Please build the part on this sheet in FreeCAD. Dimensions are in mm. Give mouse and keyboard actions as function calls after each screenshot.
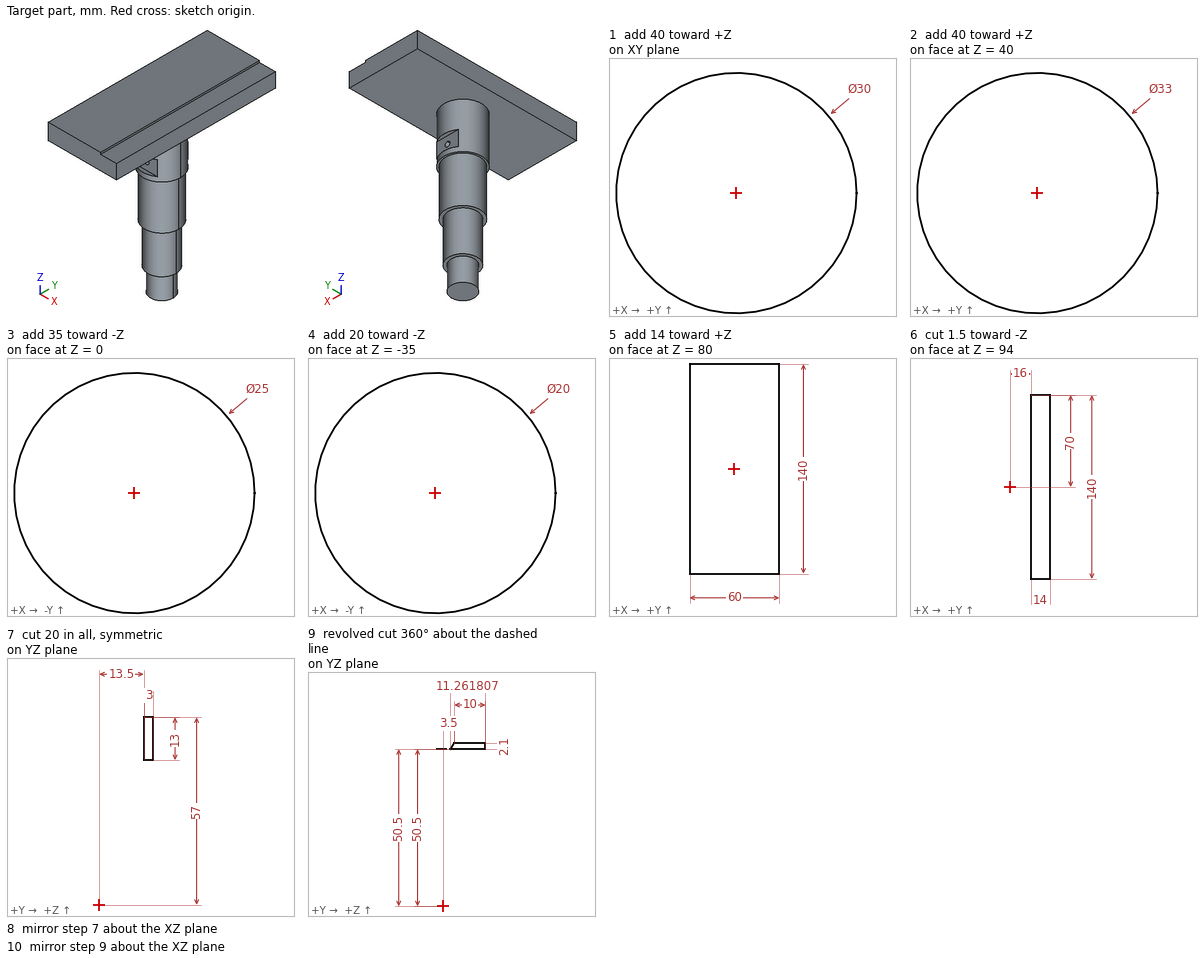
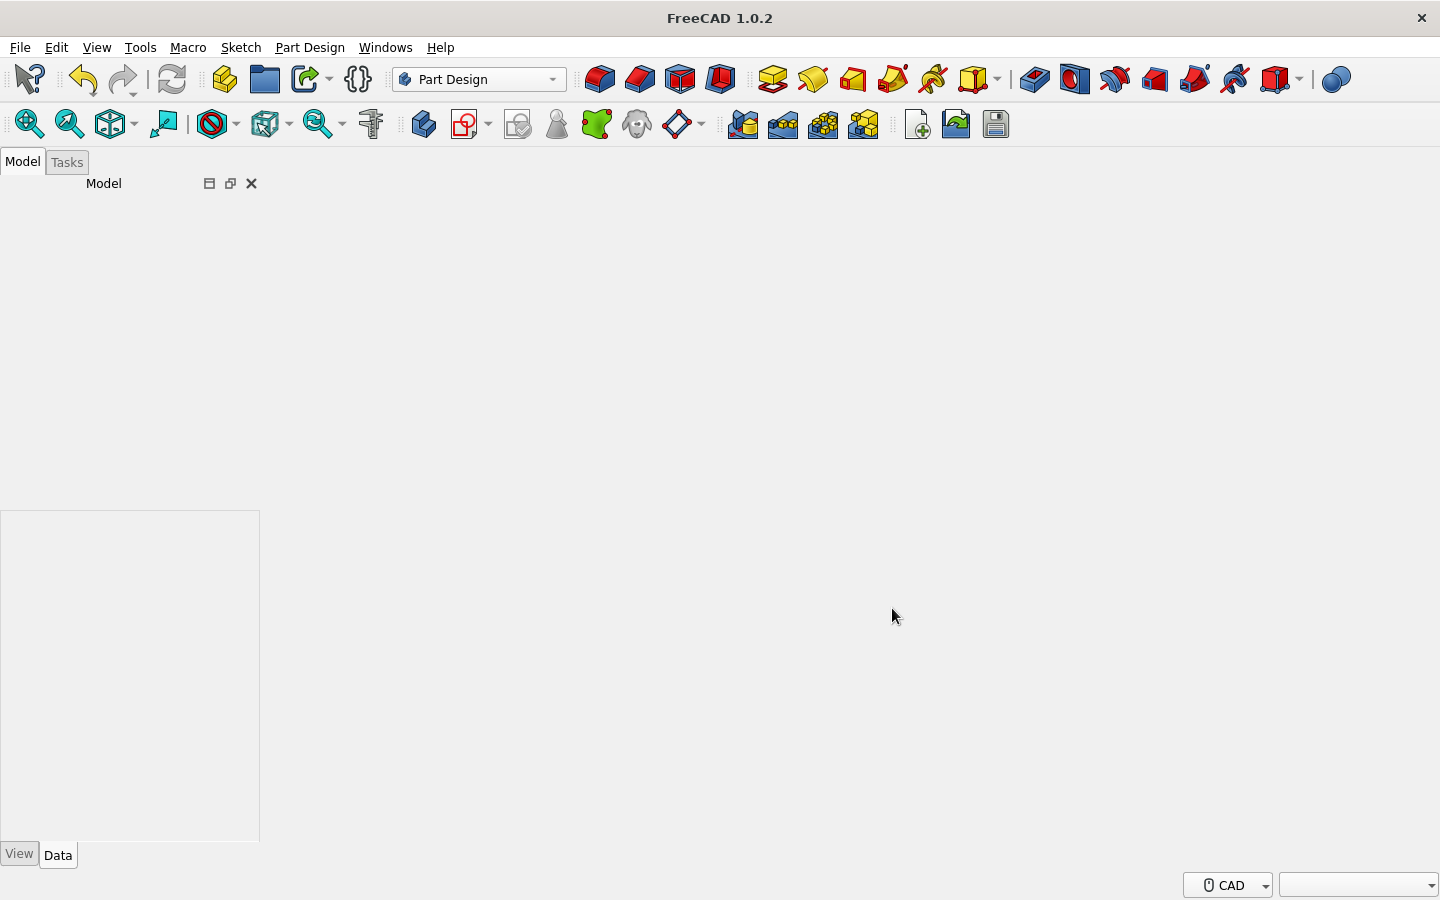
click(916, 124)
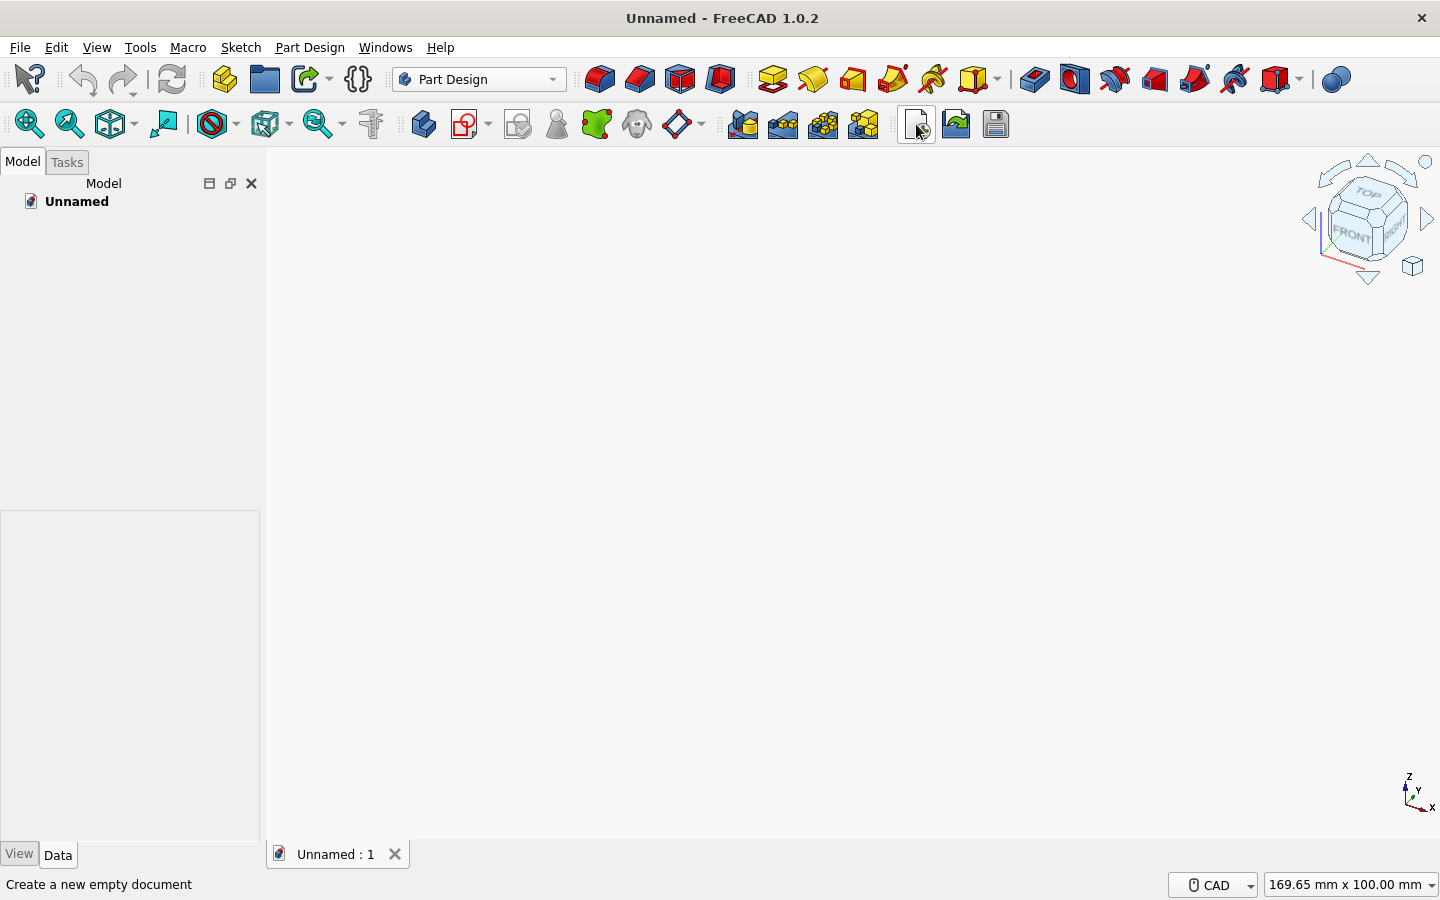
click(464, 124)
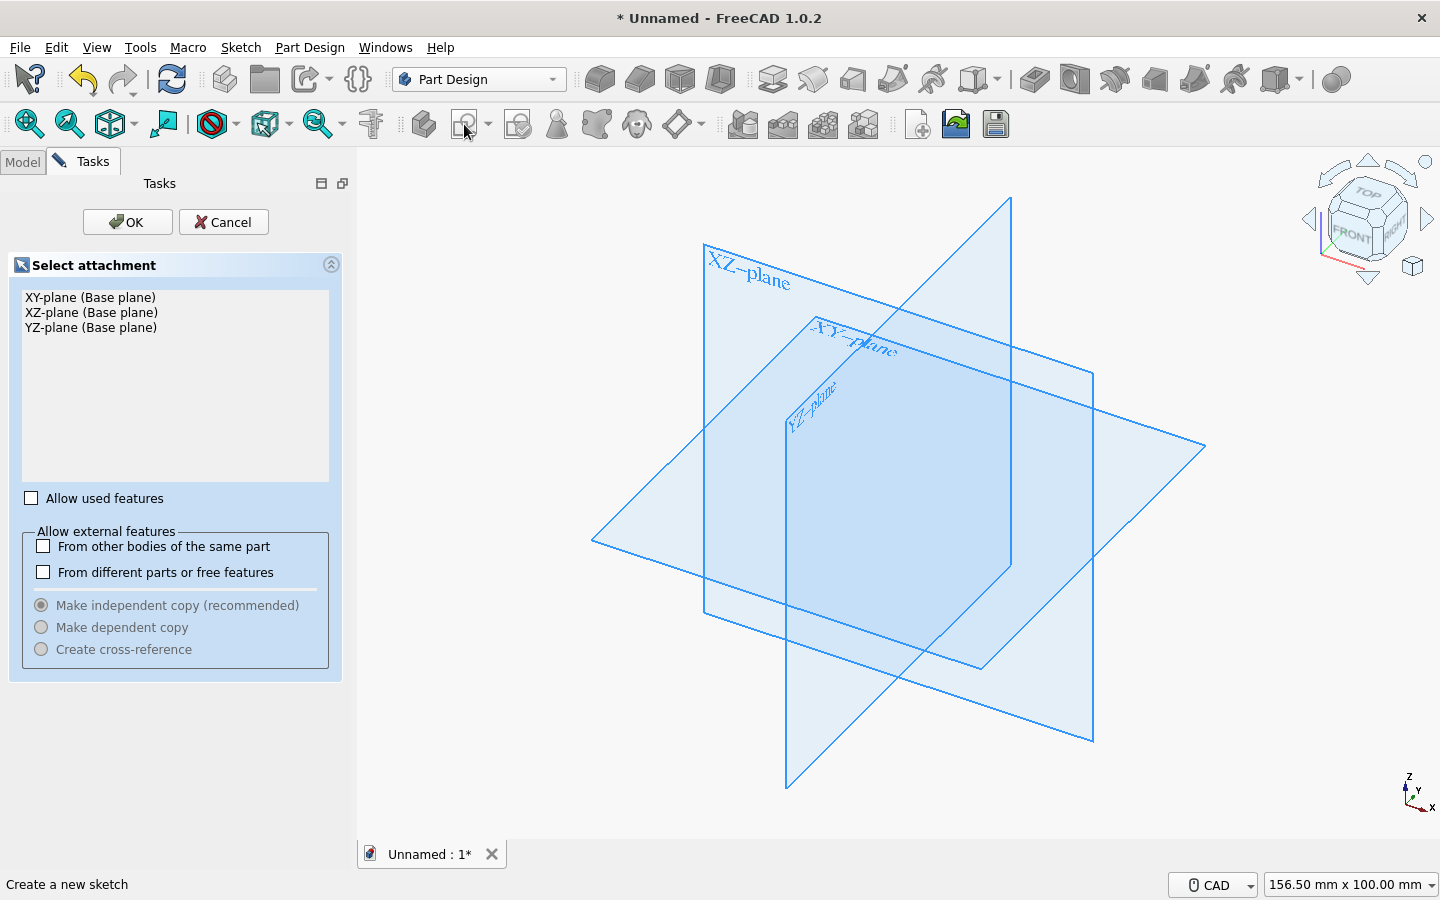
click(82, 298)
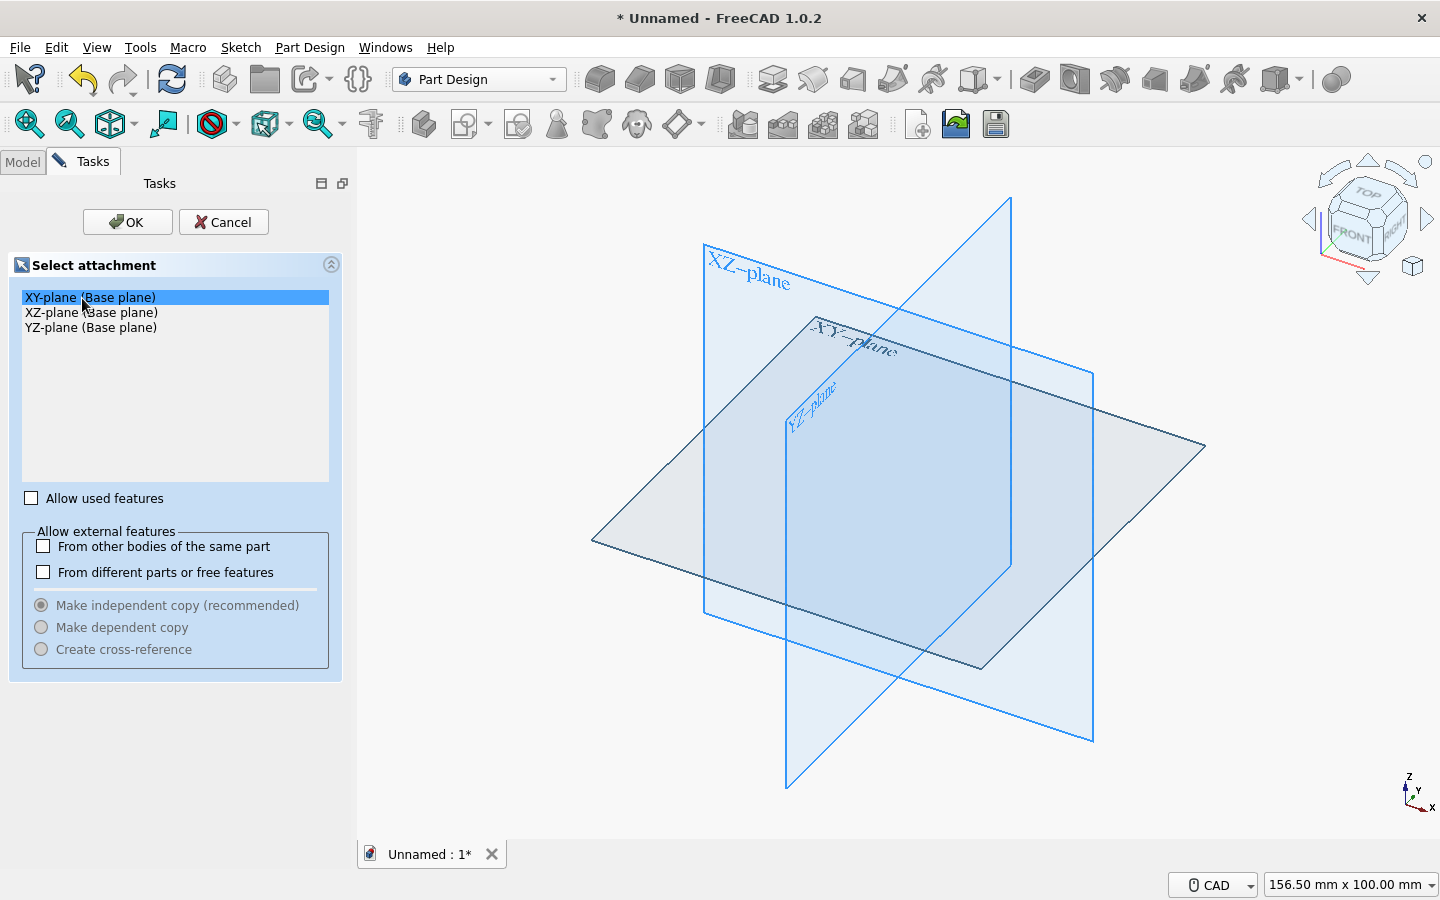
click(128, 222)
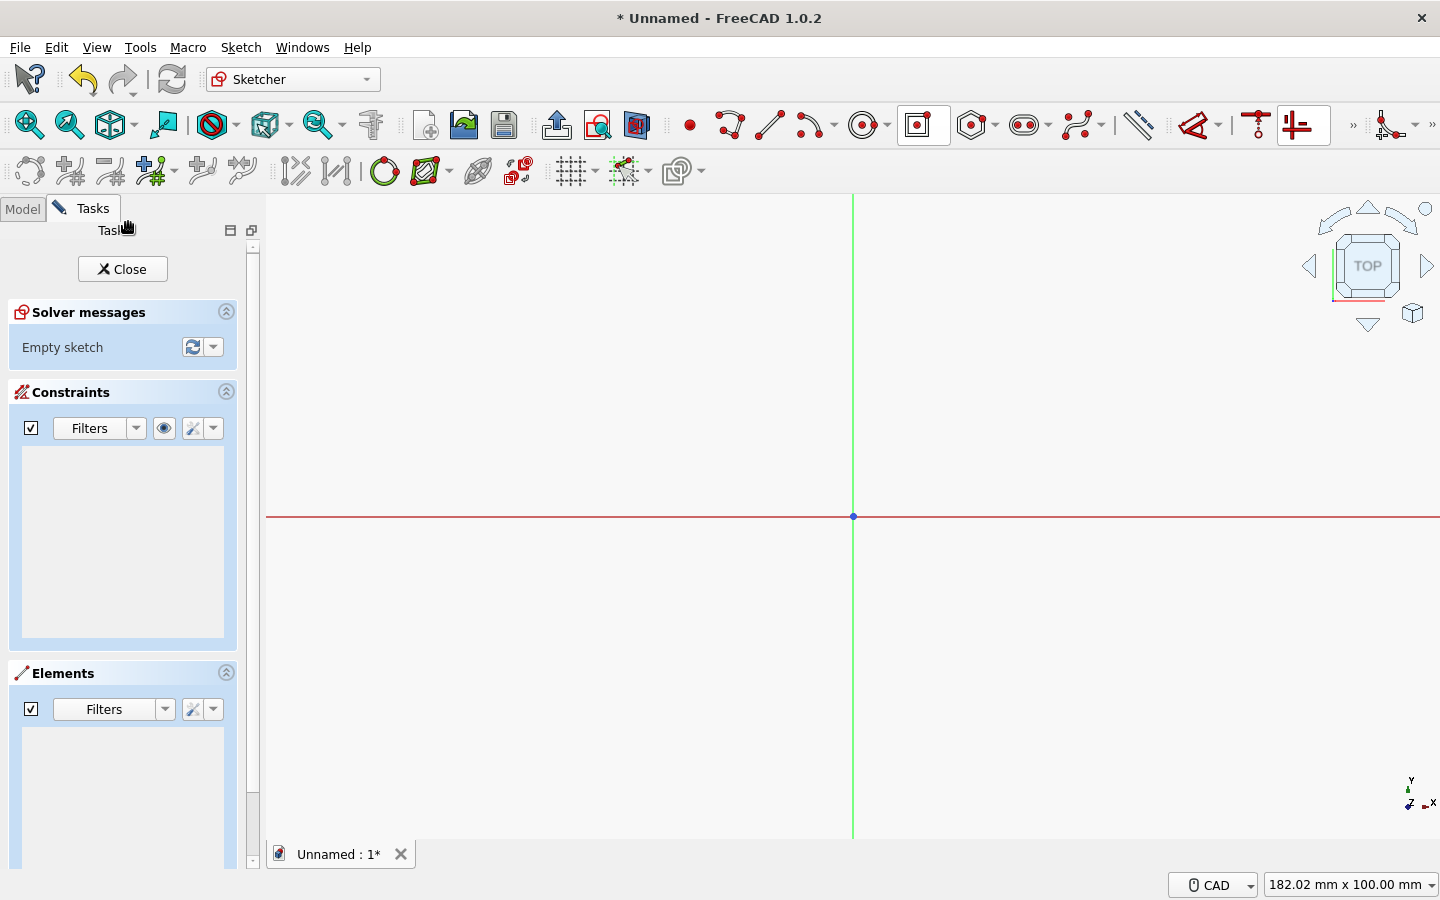
scroll(909, 517, up, 4)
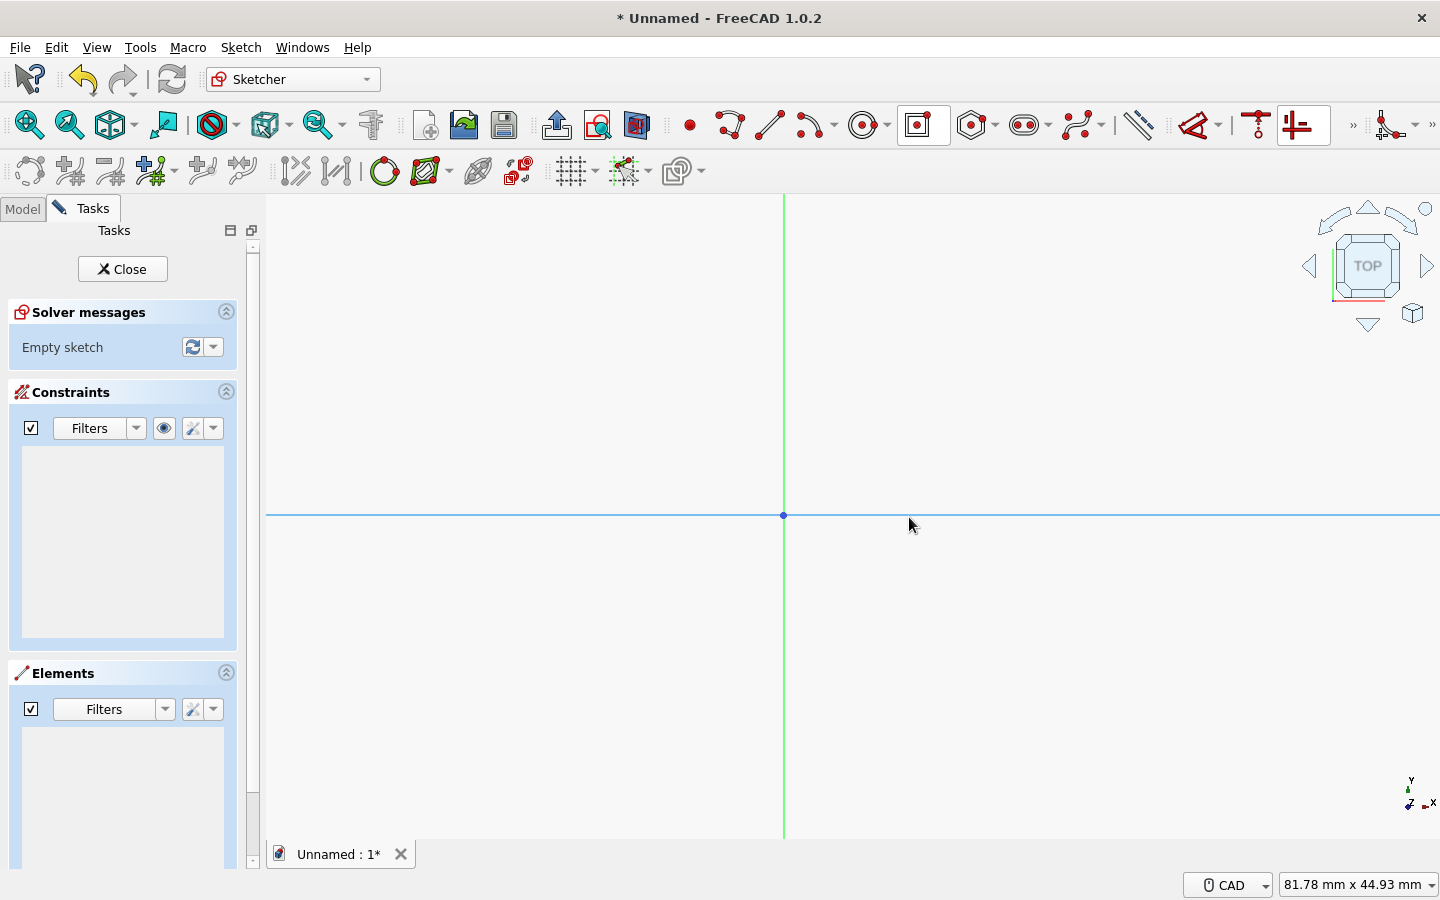
click(864, 126)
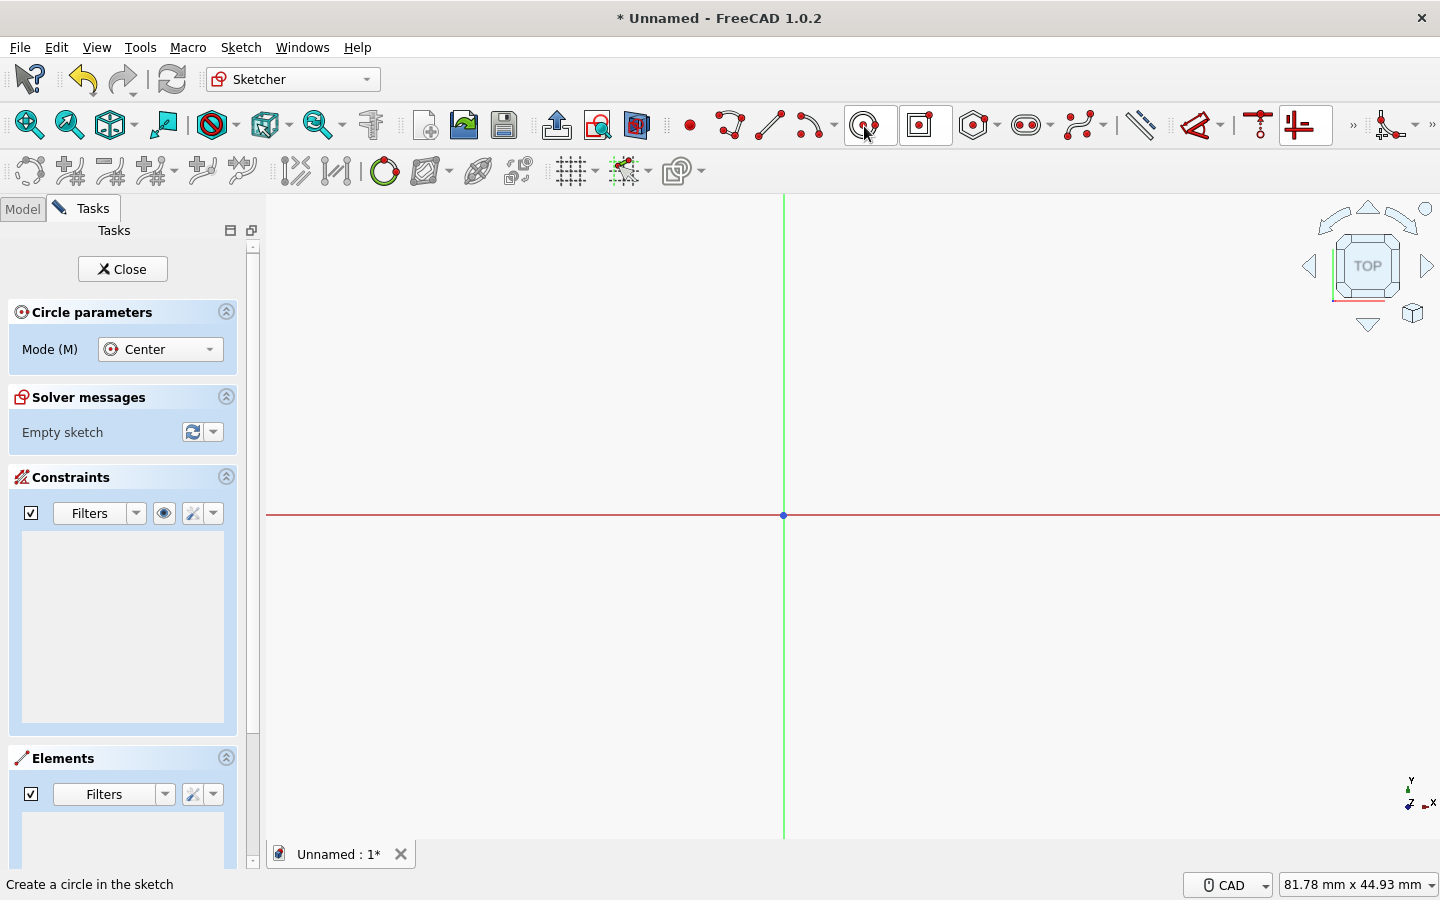
click(784, 515)
move(936, 363)